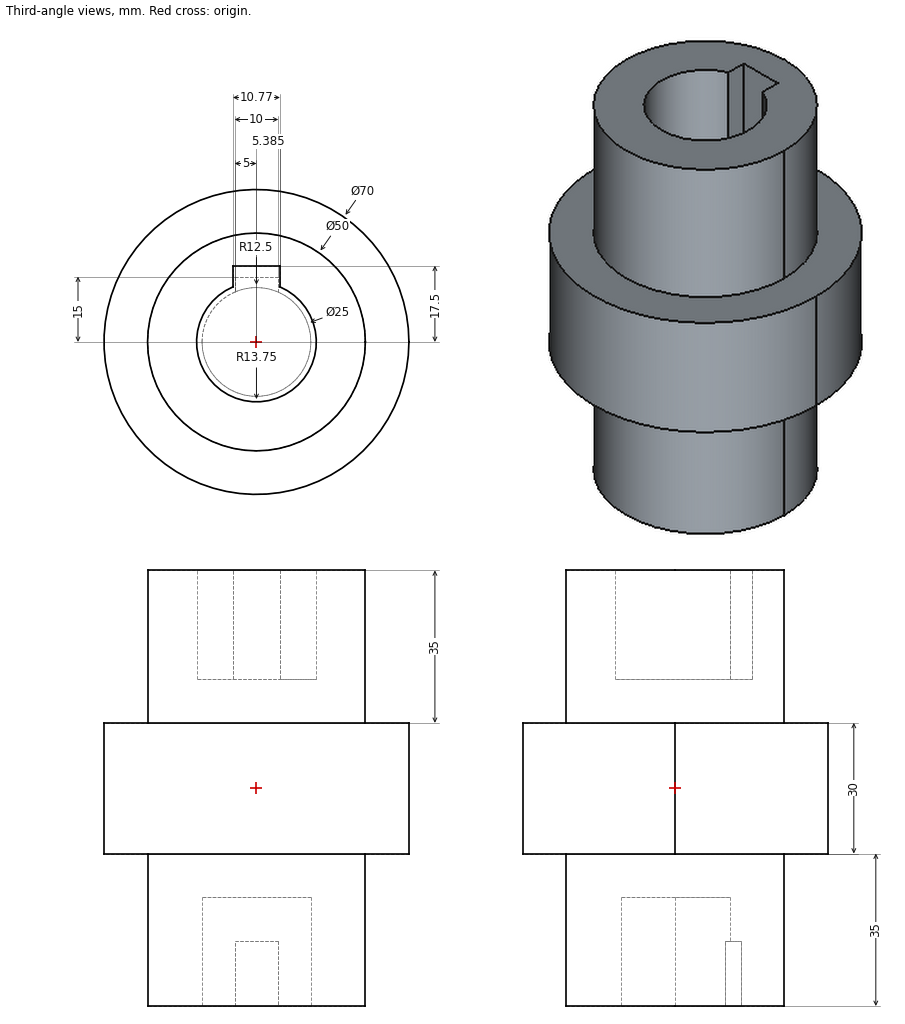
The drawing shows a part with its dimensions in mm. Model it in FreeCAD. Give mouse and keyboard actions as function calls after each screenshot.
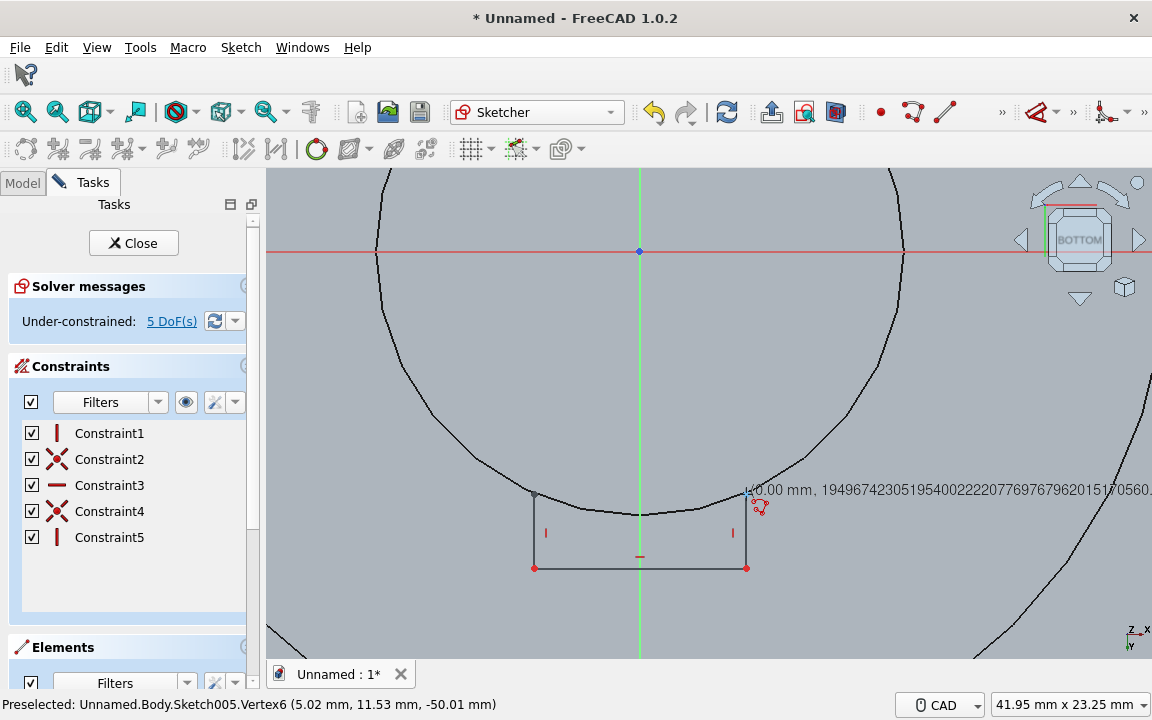
key(g)
key(3)
key(a)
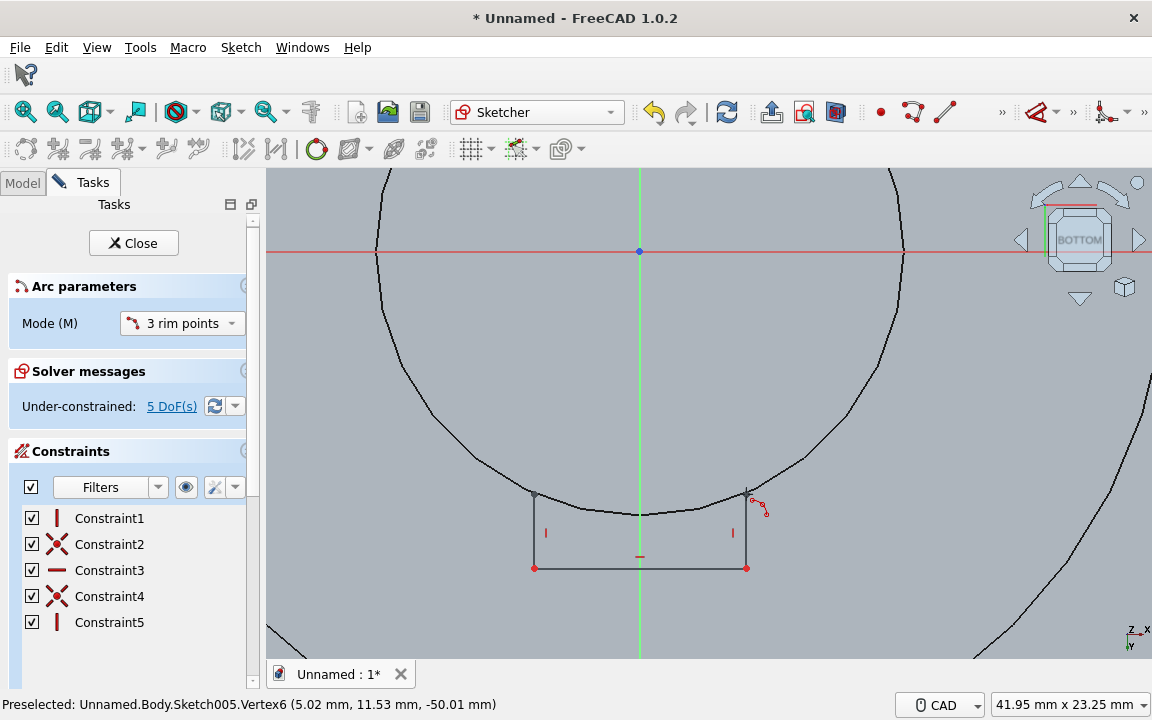
click(746, 495)
click(534, 495)
click(618, 515)
key(Escape)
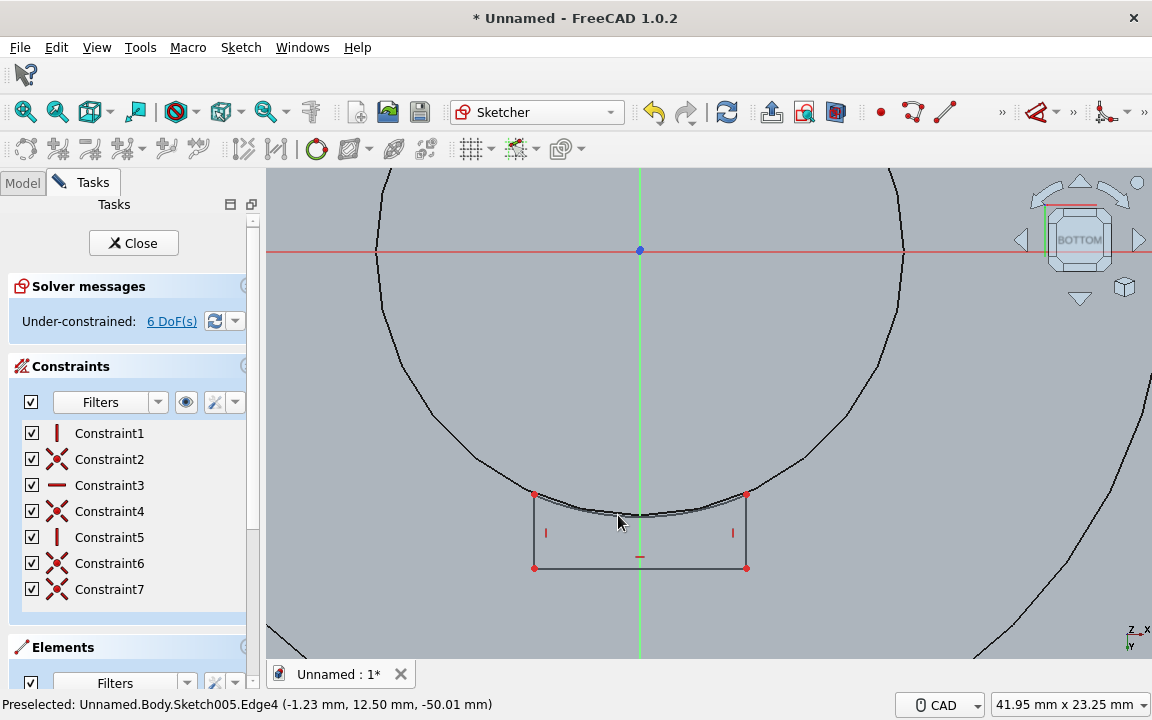
drag(630, 239, 650, 262)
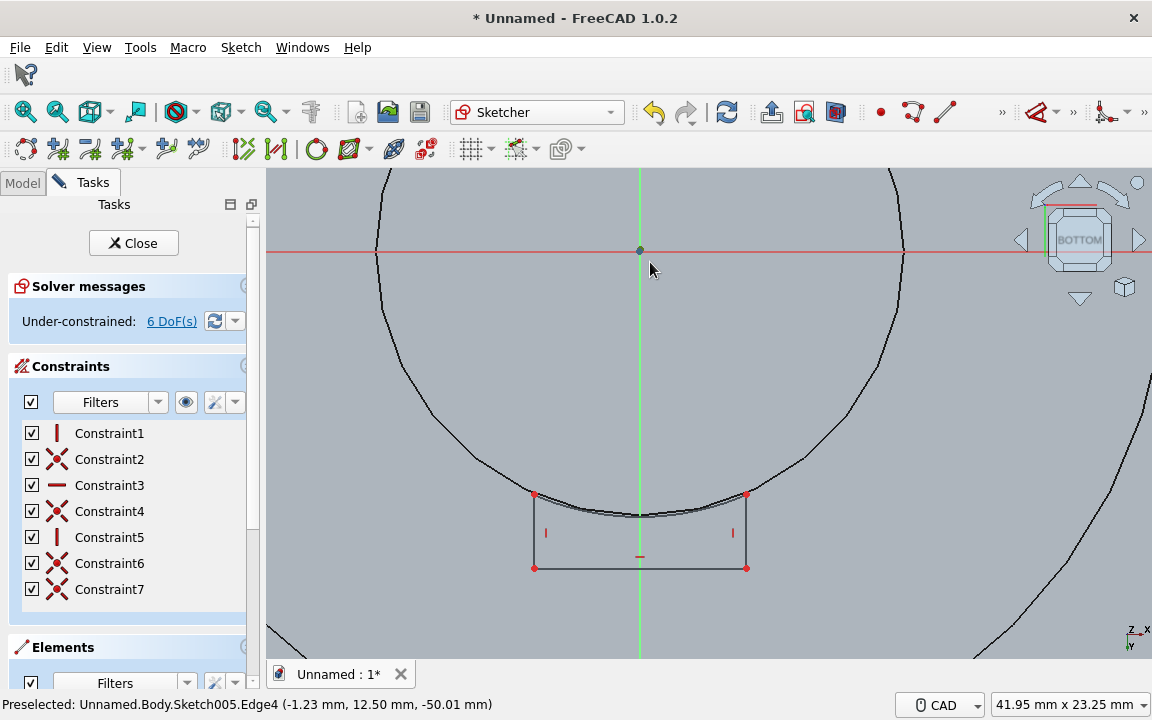
key(c)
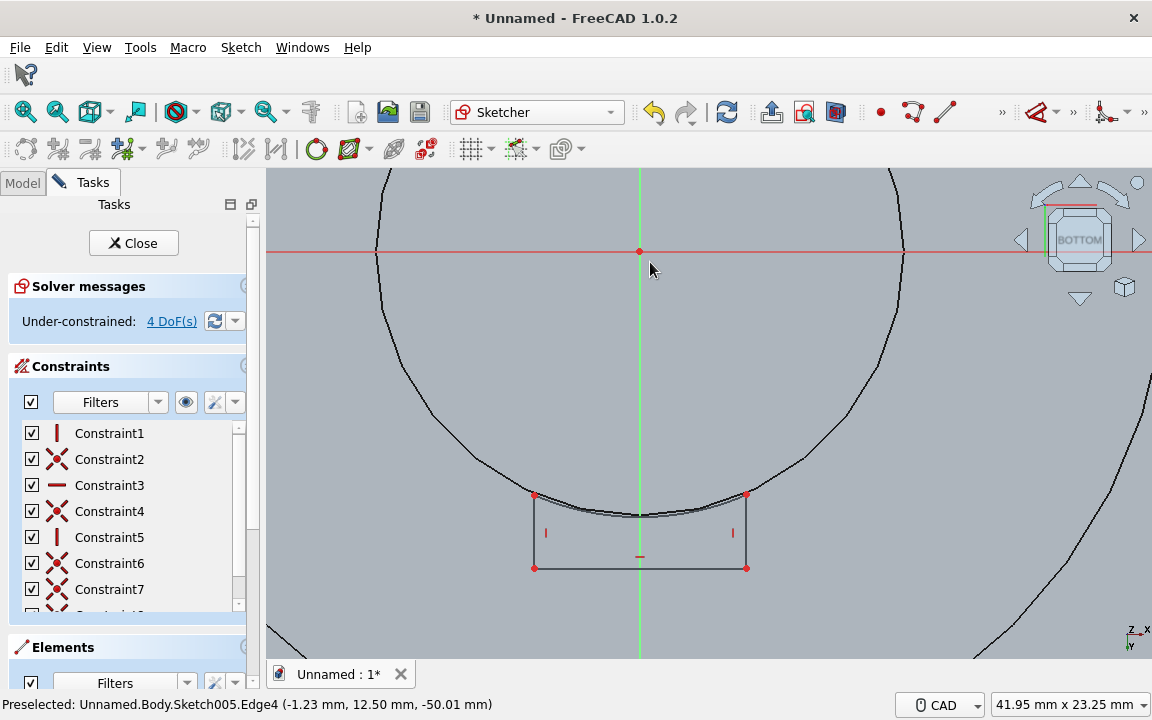
click(1036, 112)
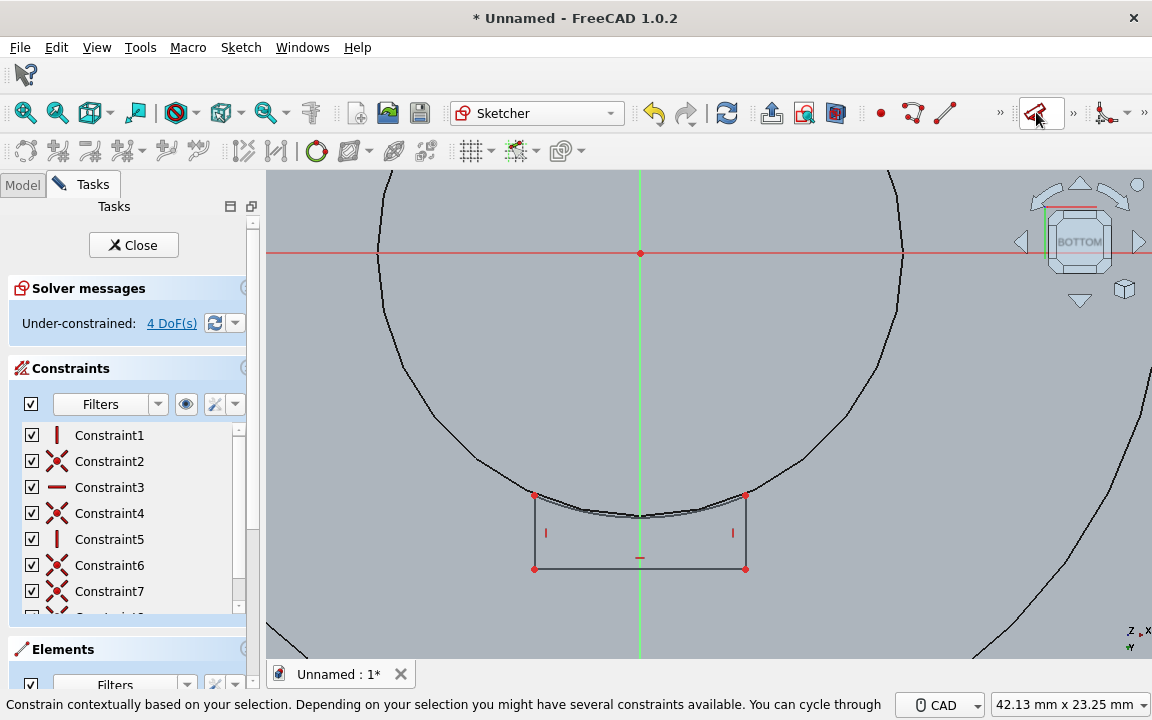
click(597, 514)
click(592, 546)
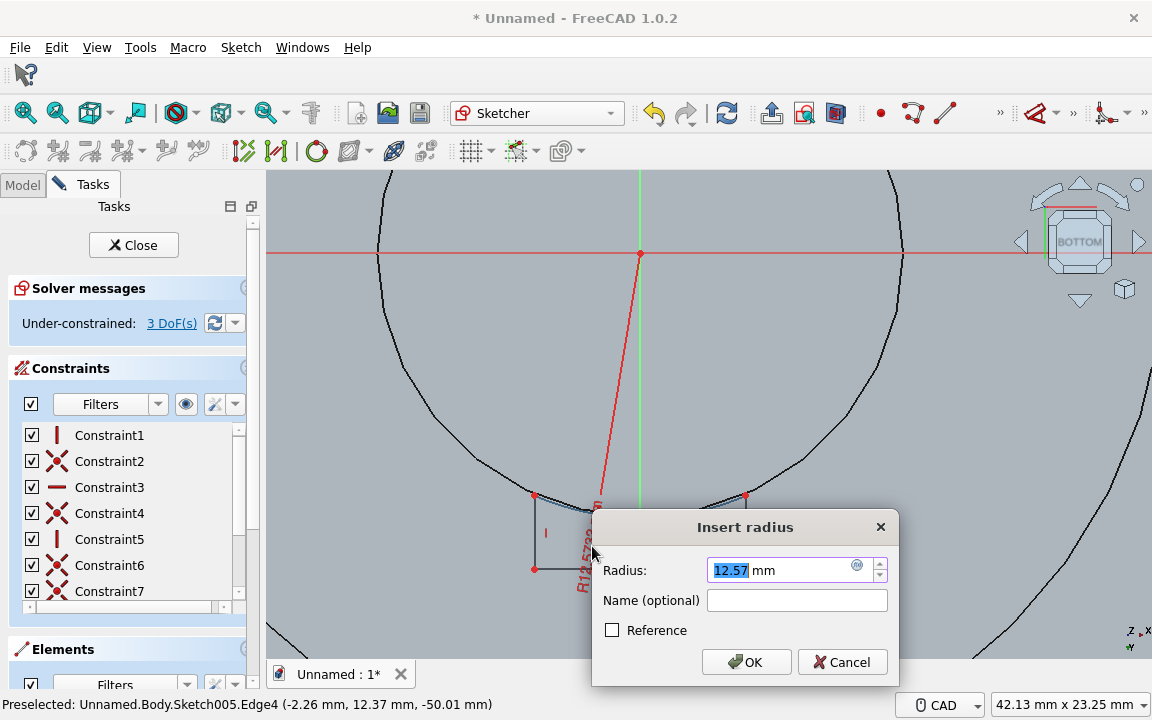
text(12.5)
key(Return)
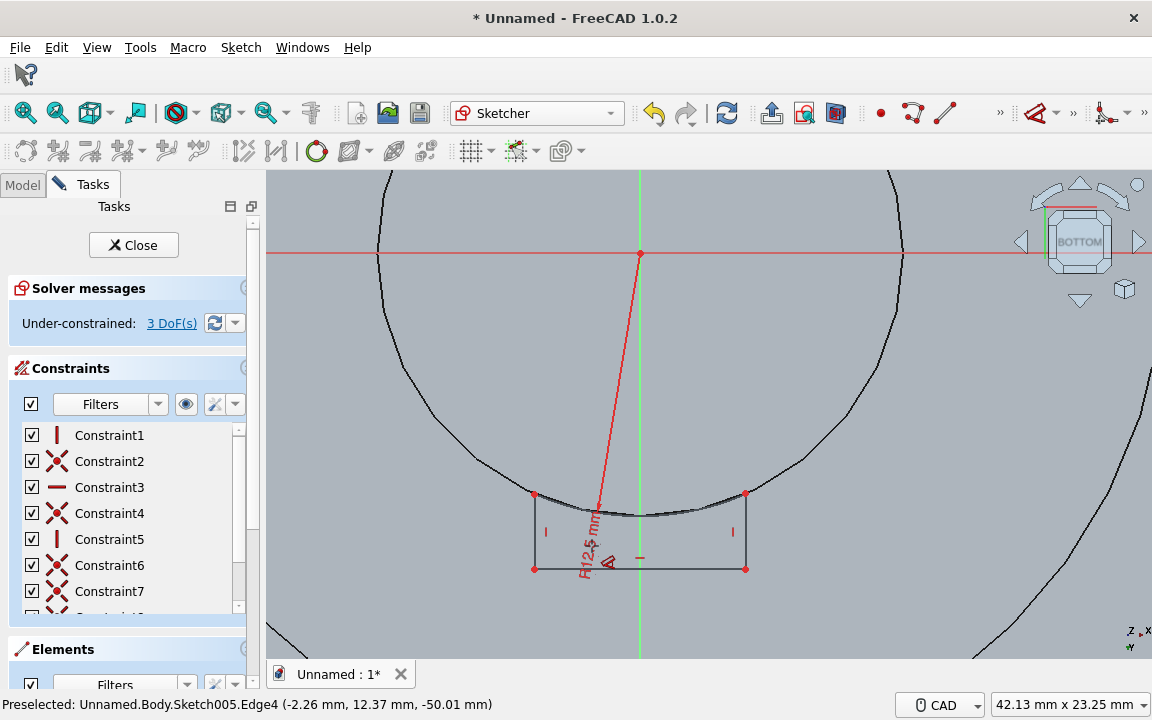
click(598, 569)
click(592, 603)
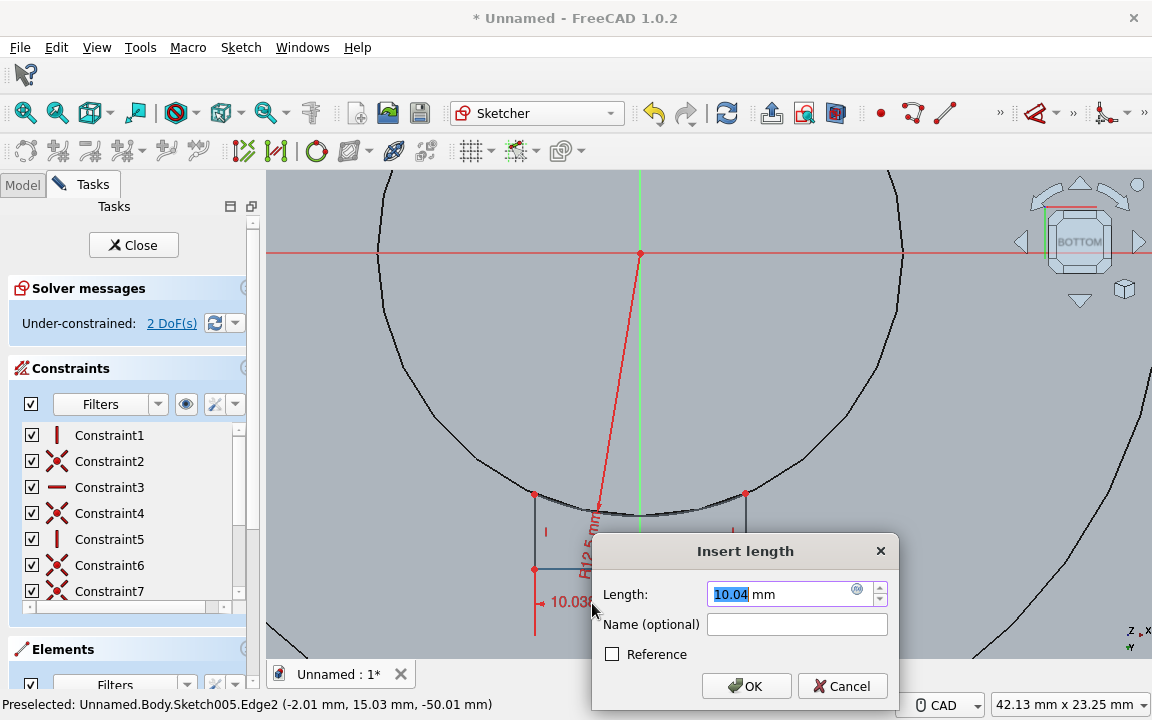
text(10)
key(Return)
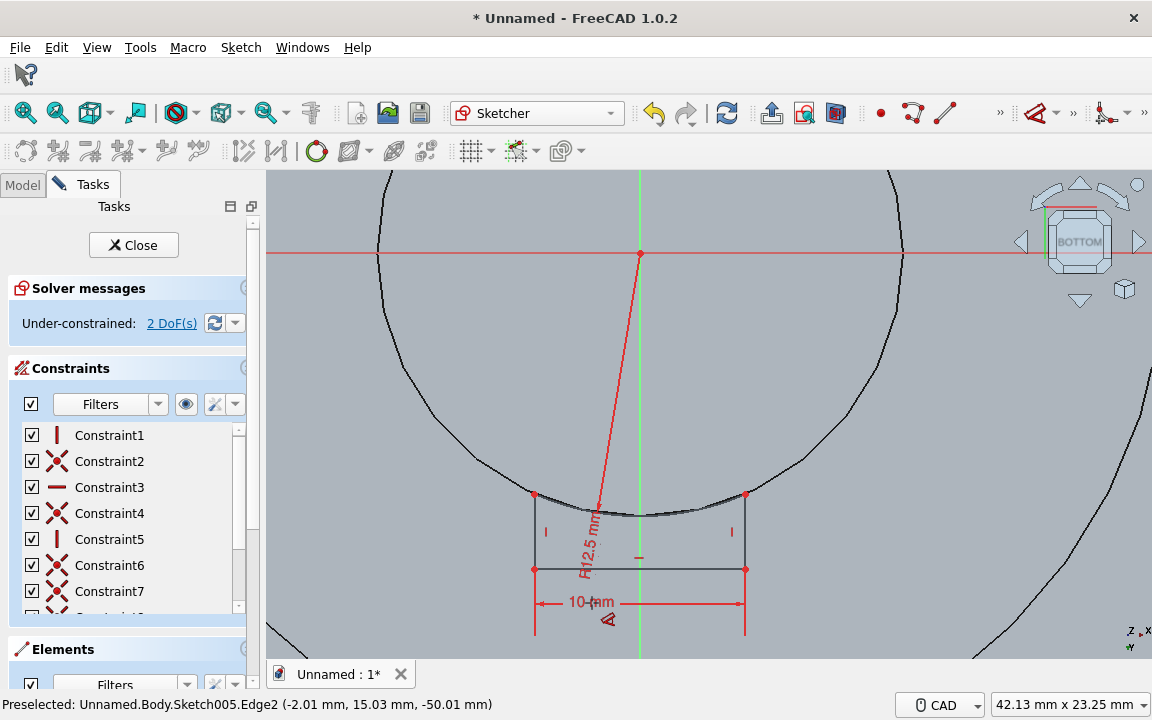
click(535, 494)
click(587, 219)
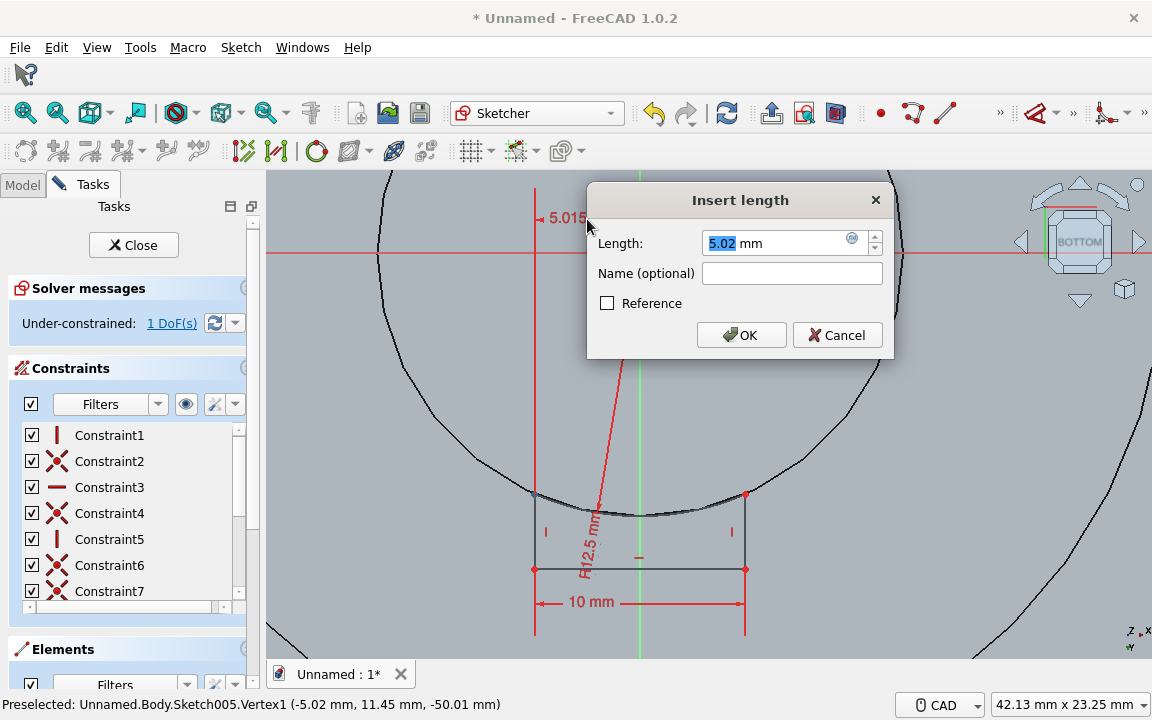
text(5)
key(Return)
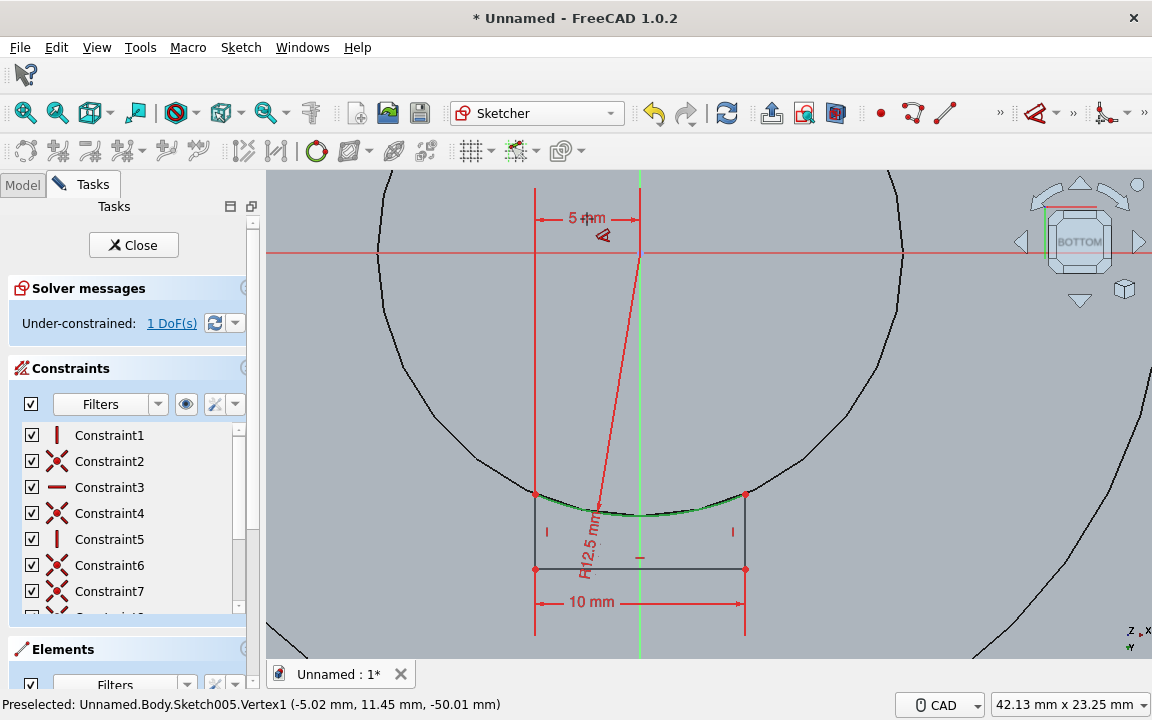
click(535, 569)
click(501, 411)